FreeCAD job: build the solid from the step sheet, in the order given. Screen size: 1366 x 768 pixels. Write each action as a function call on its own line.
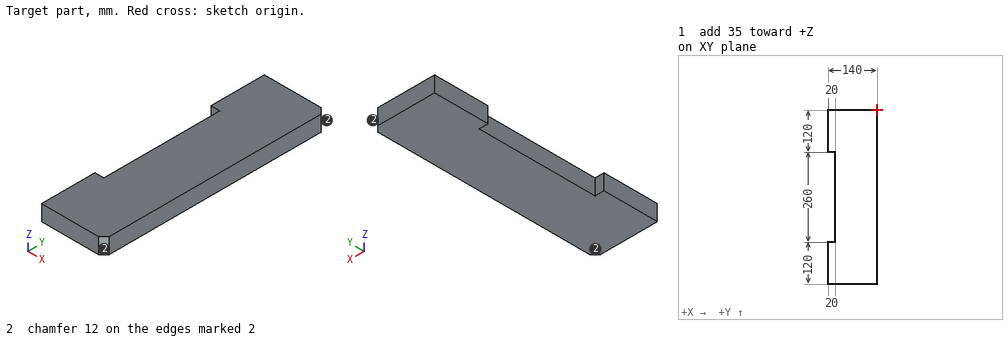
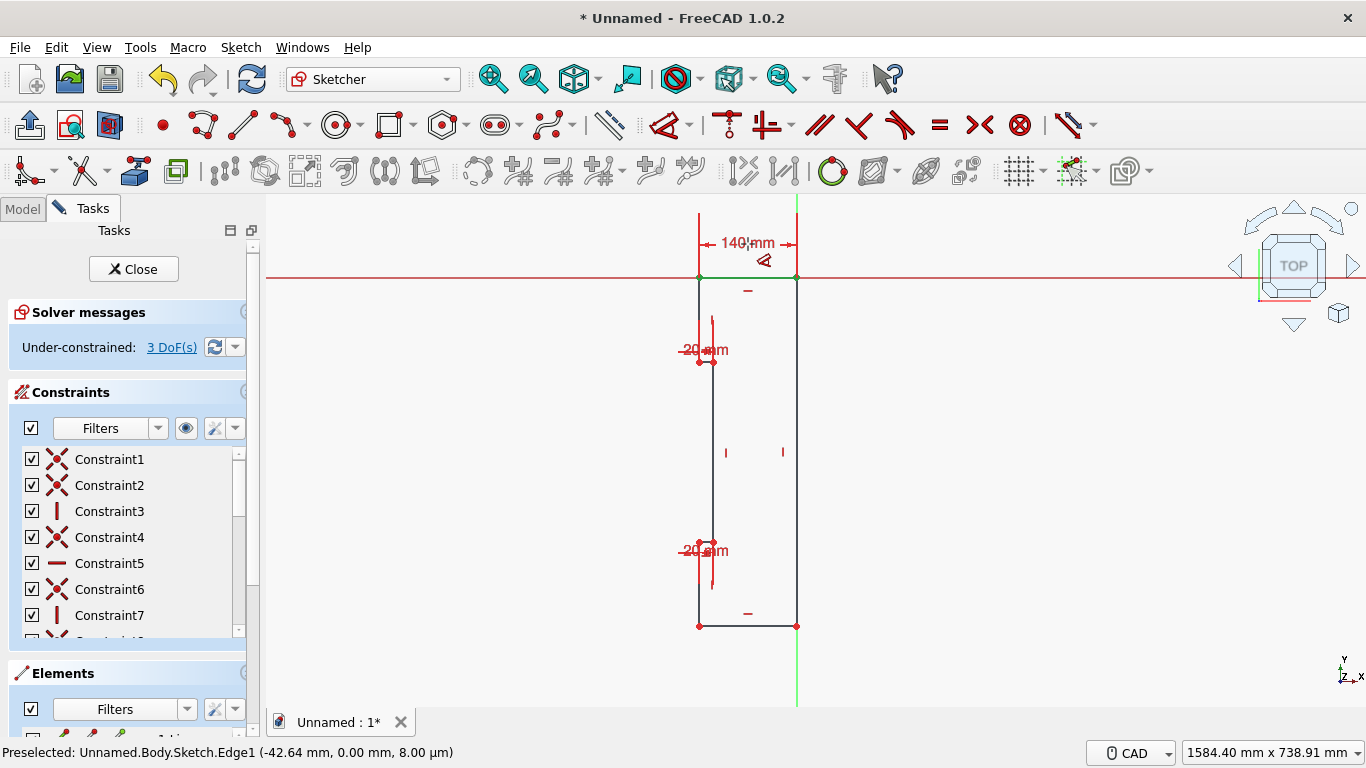
click(699, 303)
click(665, 320)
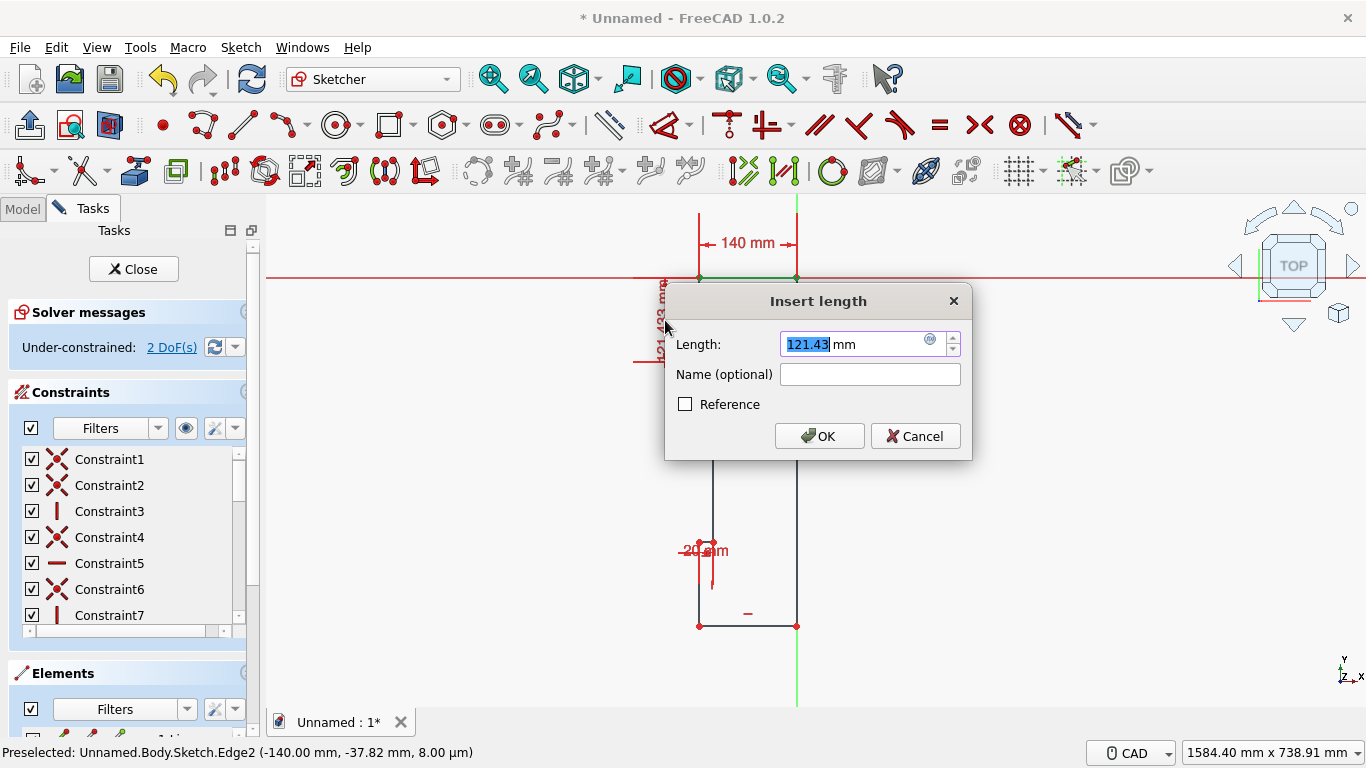
text(120)
key(Return)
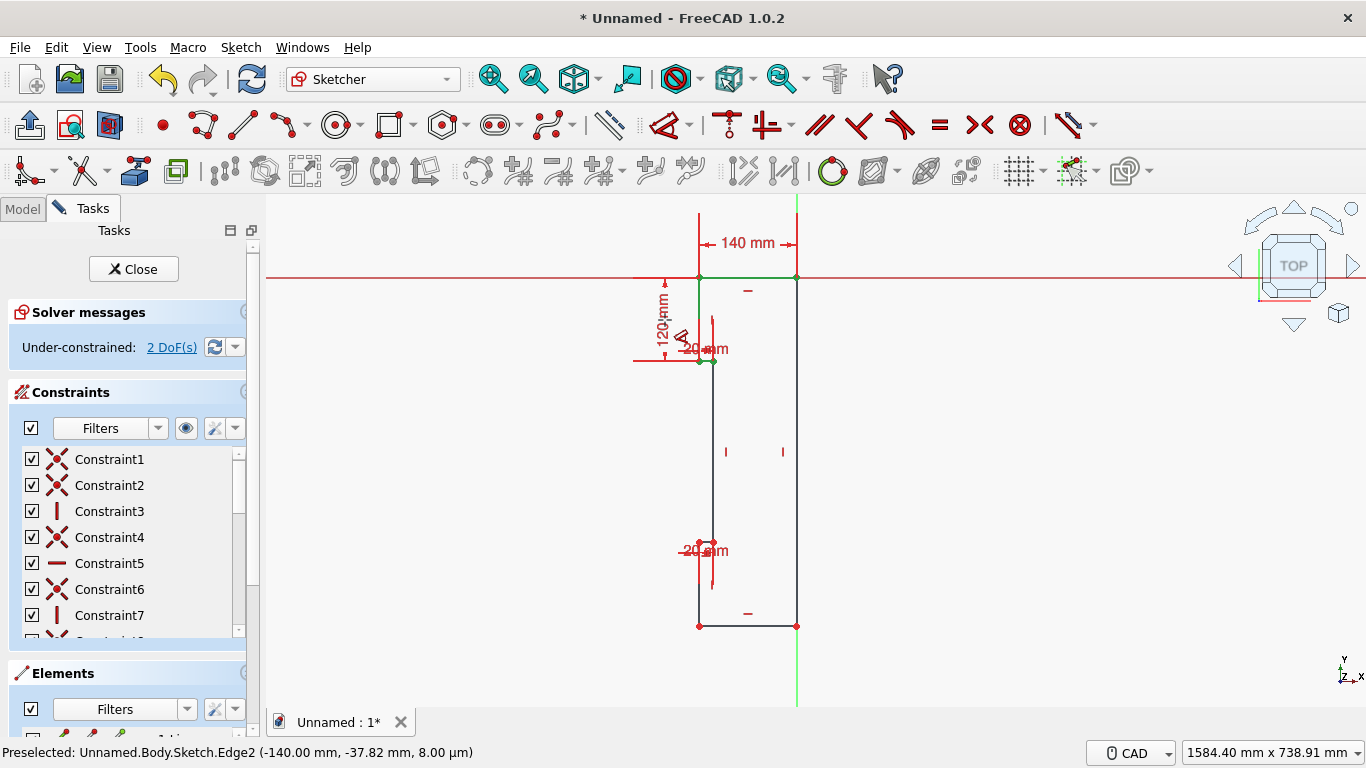
click(713, 415)
click(679, 452)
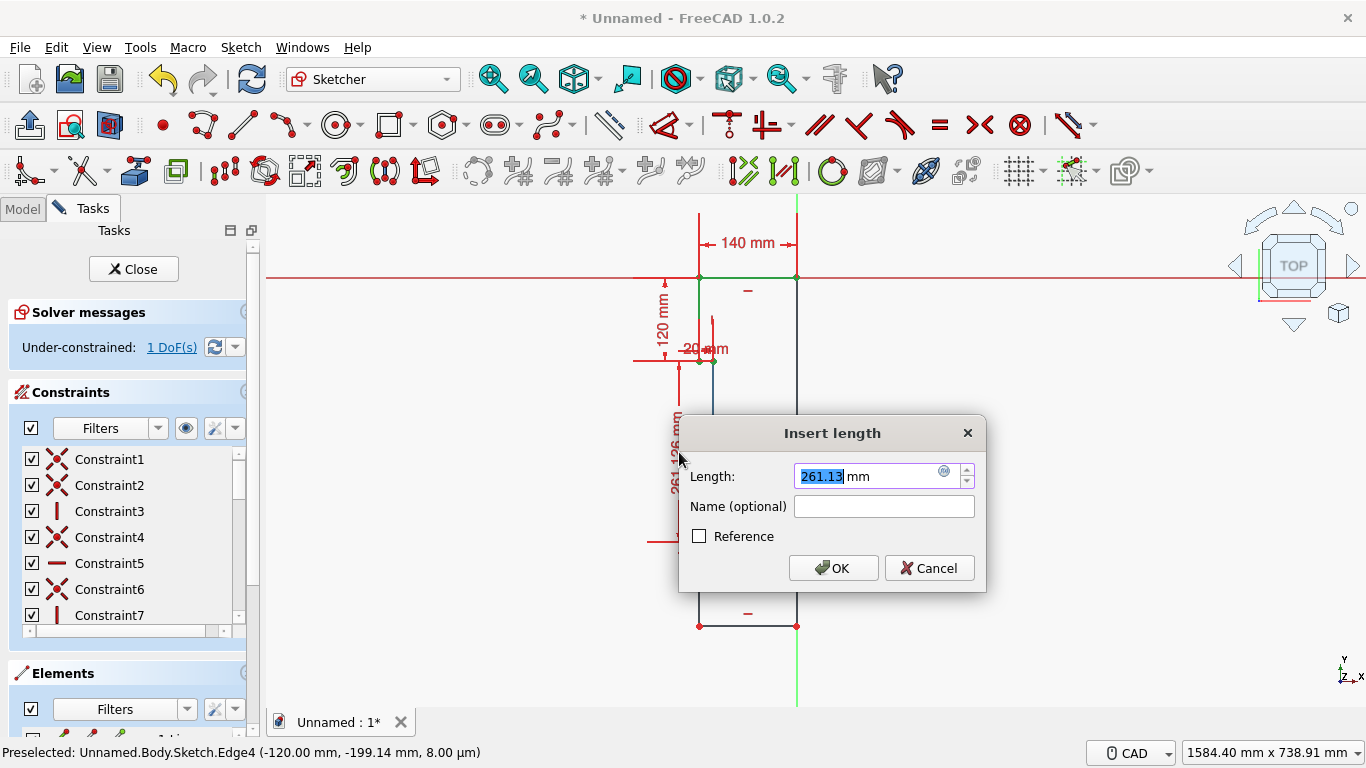
text(260)
key(Return)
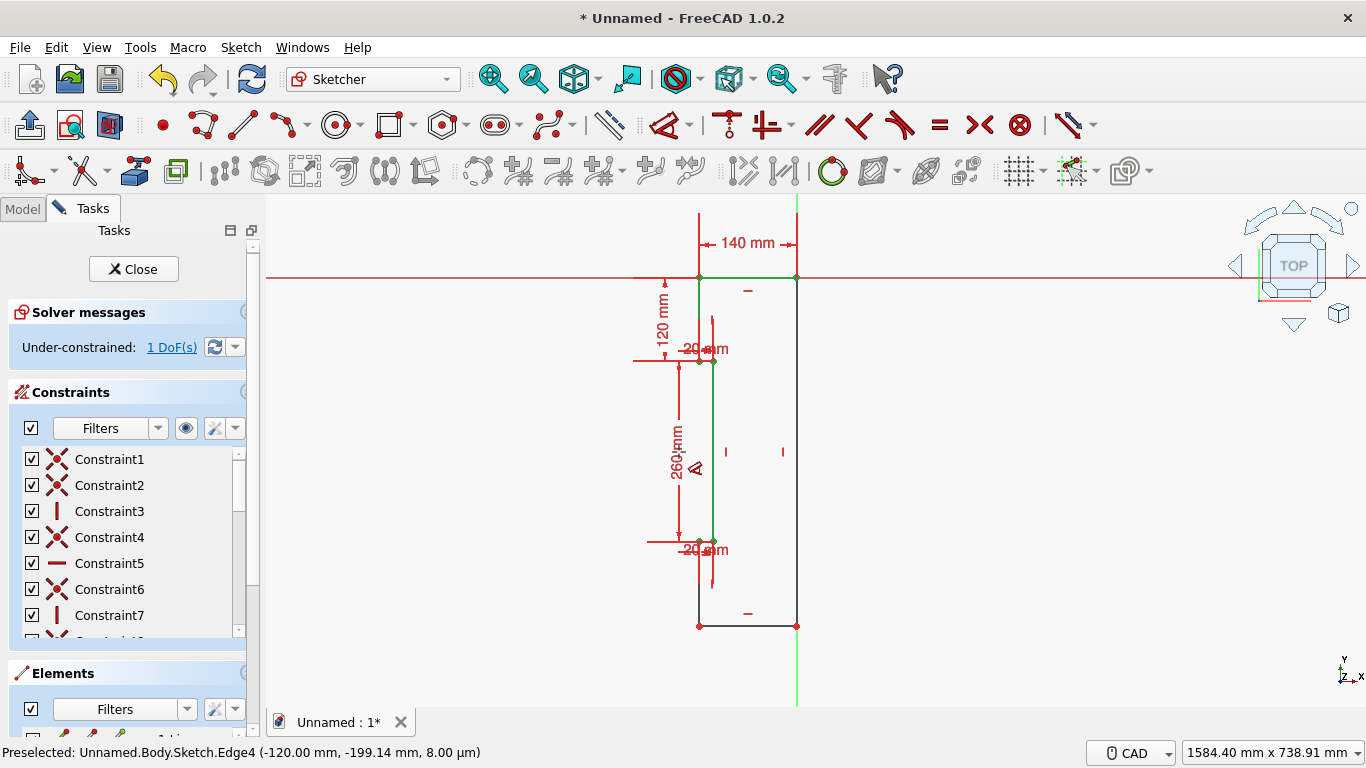
click(699, 567)
click(665, 584)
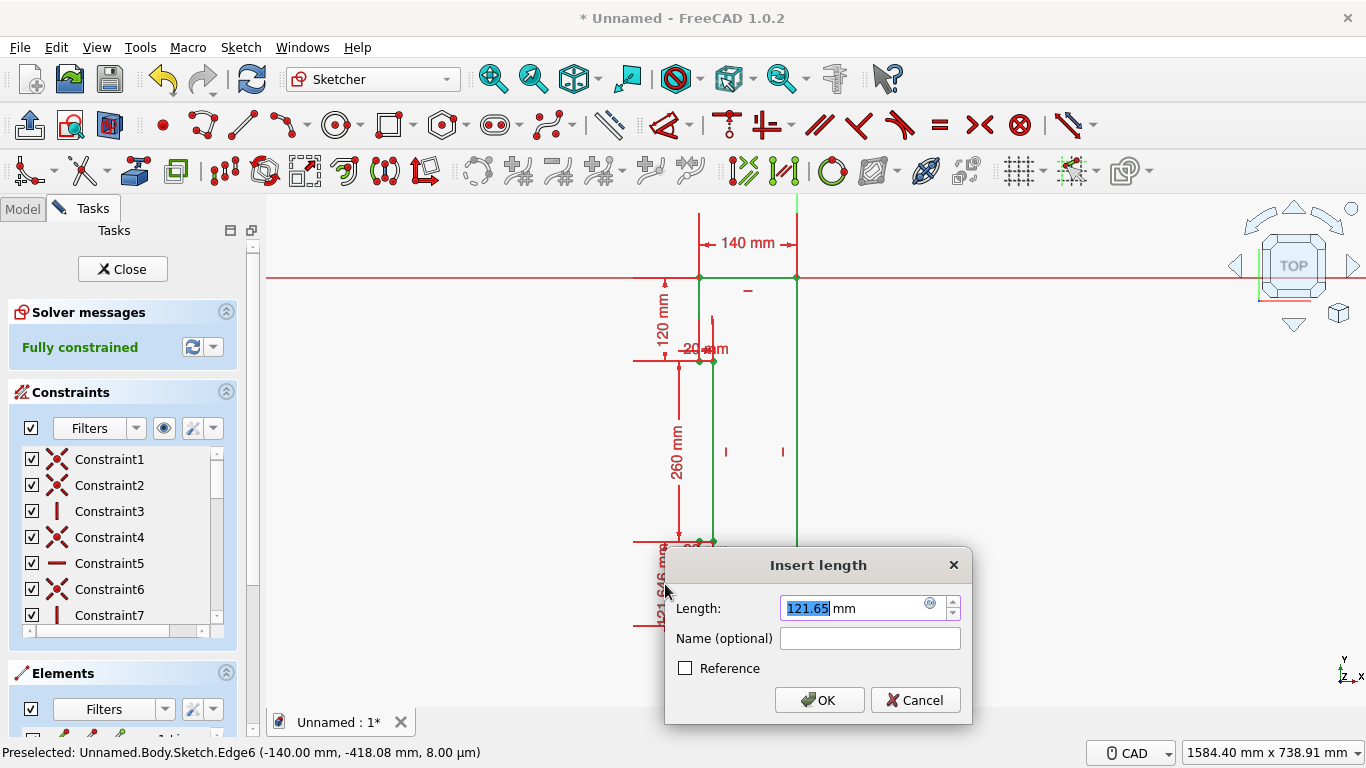
text(120)
key(Return)
key(Escape)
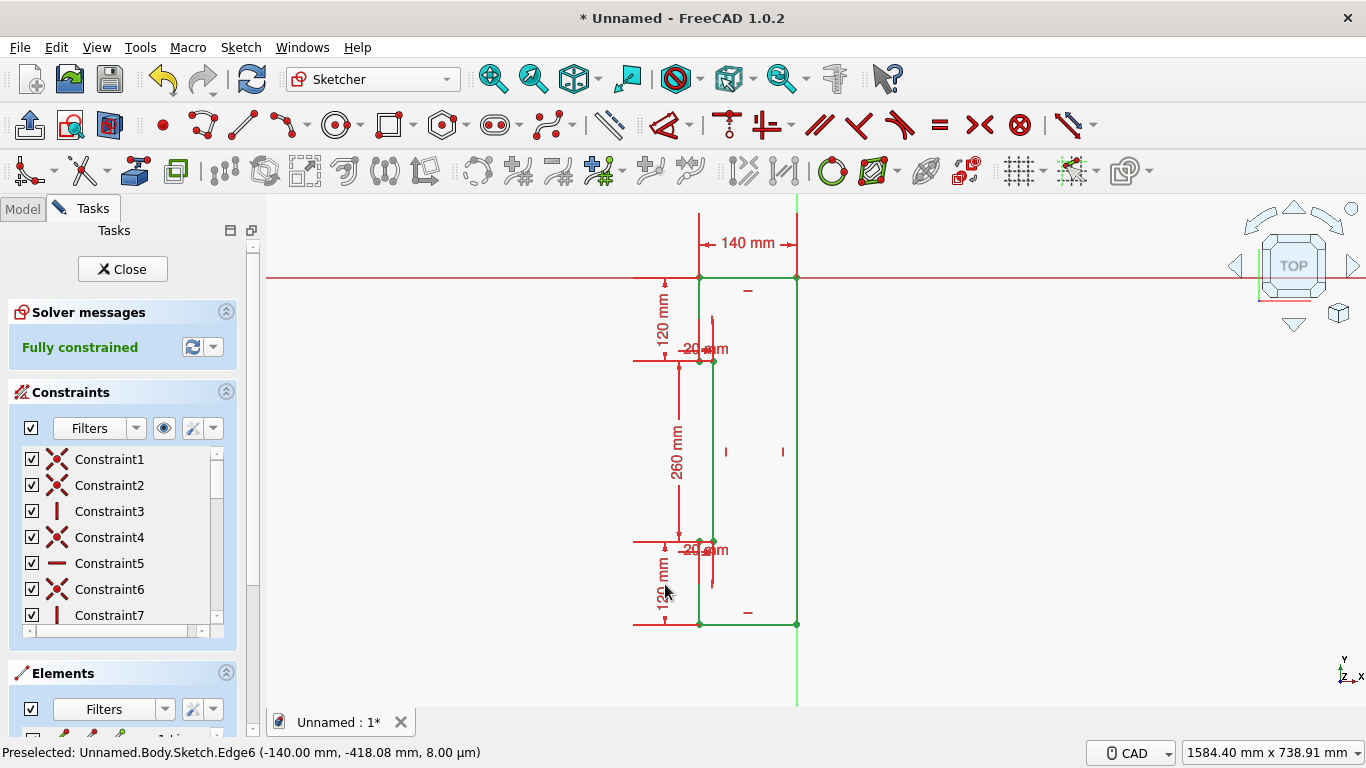
click(123, 269)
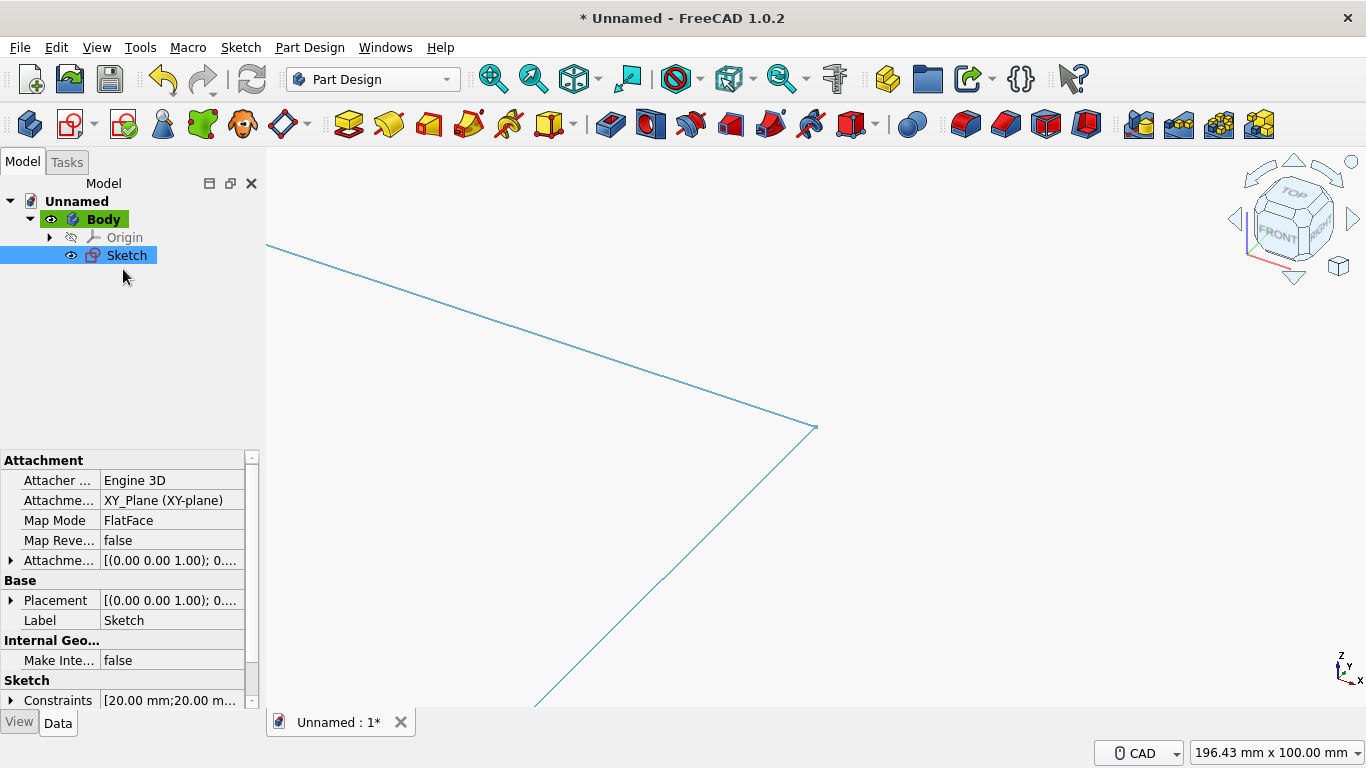
click(350, 124)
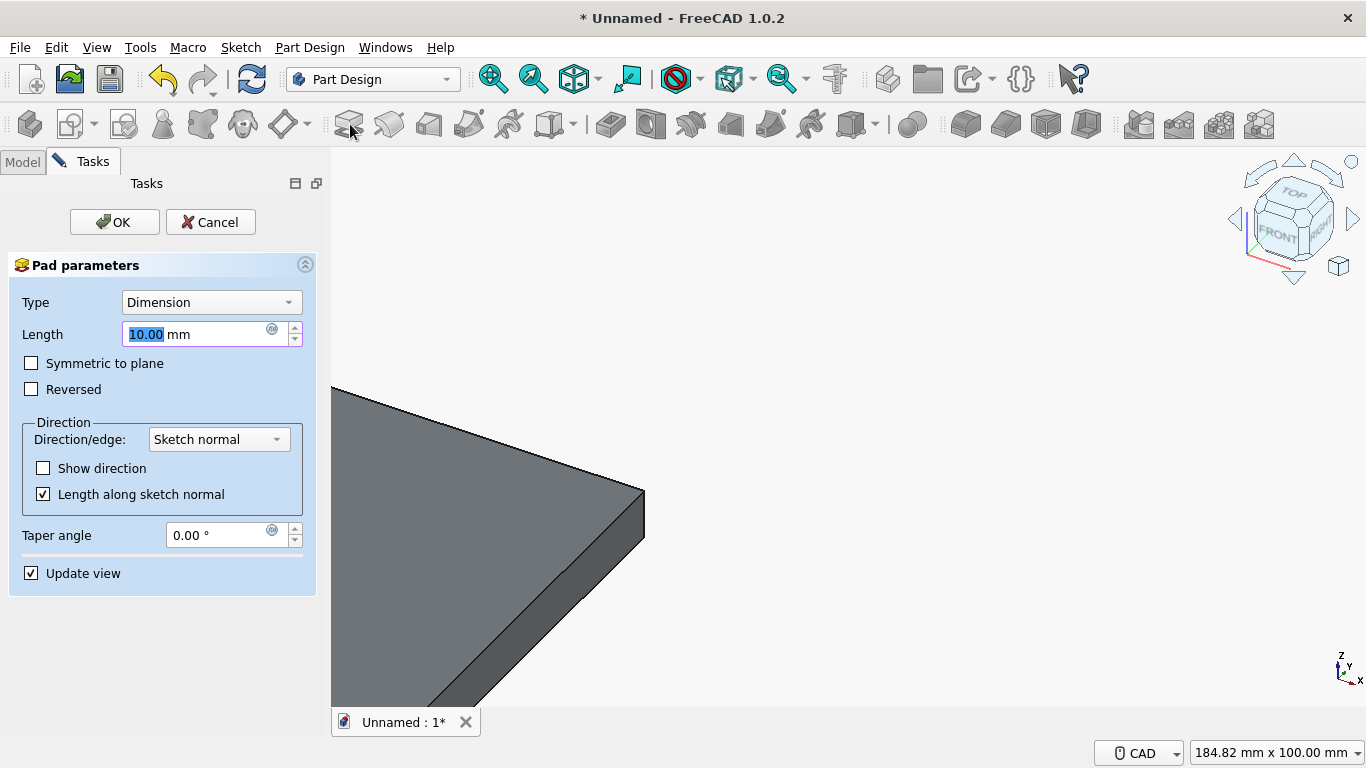
text(35)
key(Tab)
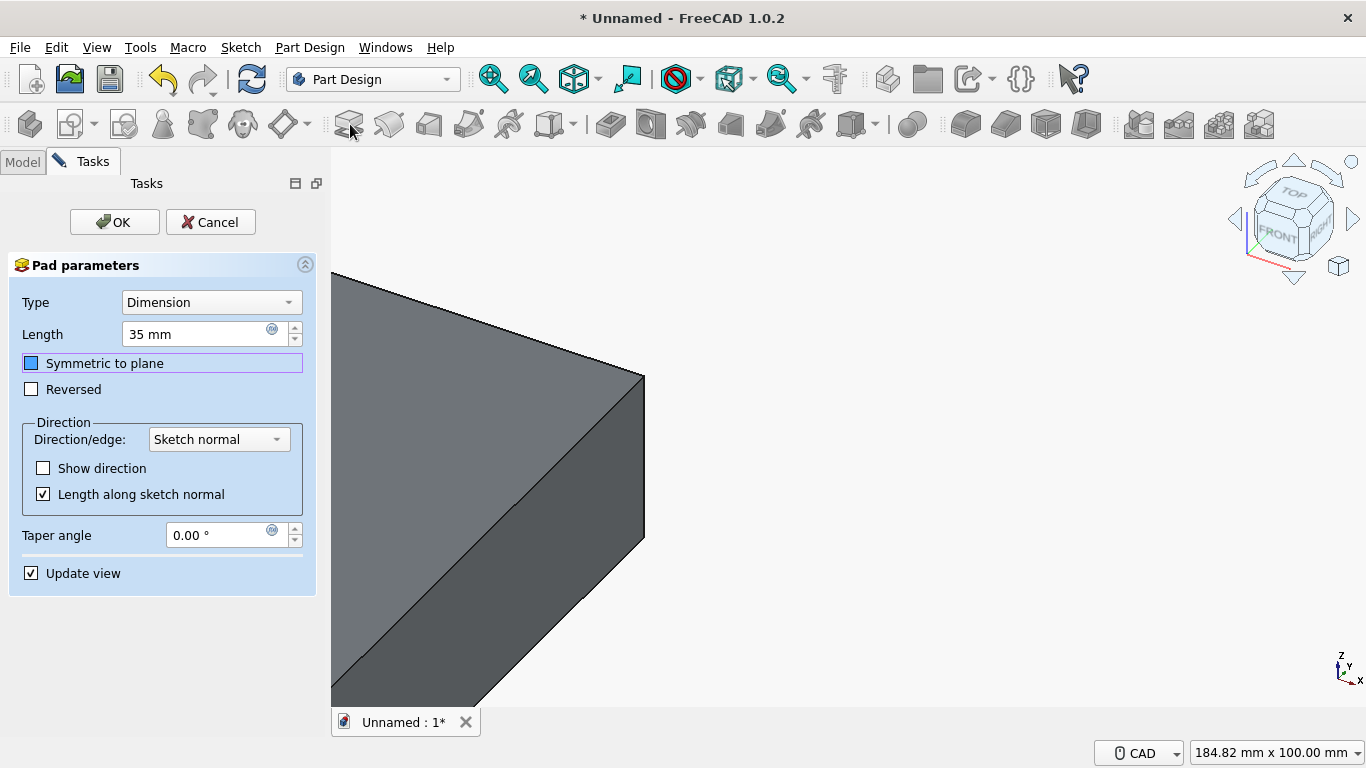
click(115, 222)